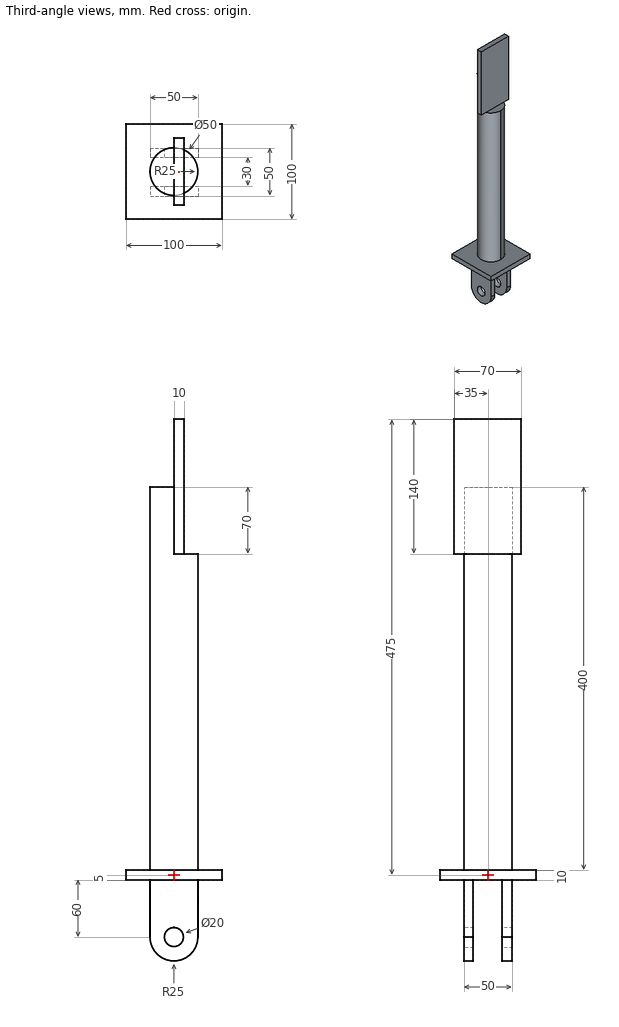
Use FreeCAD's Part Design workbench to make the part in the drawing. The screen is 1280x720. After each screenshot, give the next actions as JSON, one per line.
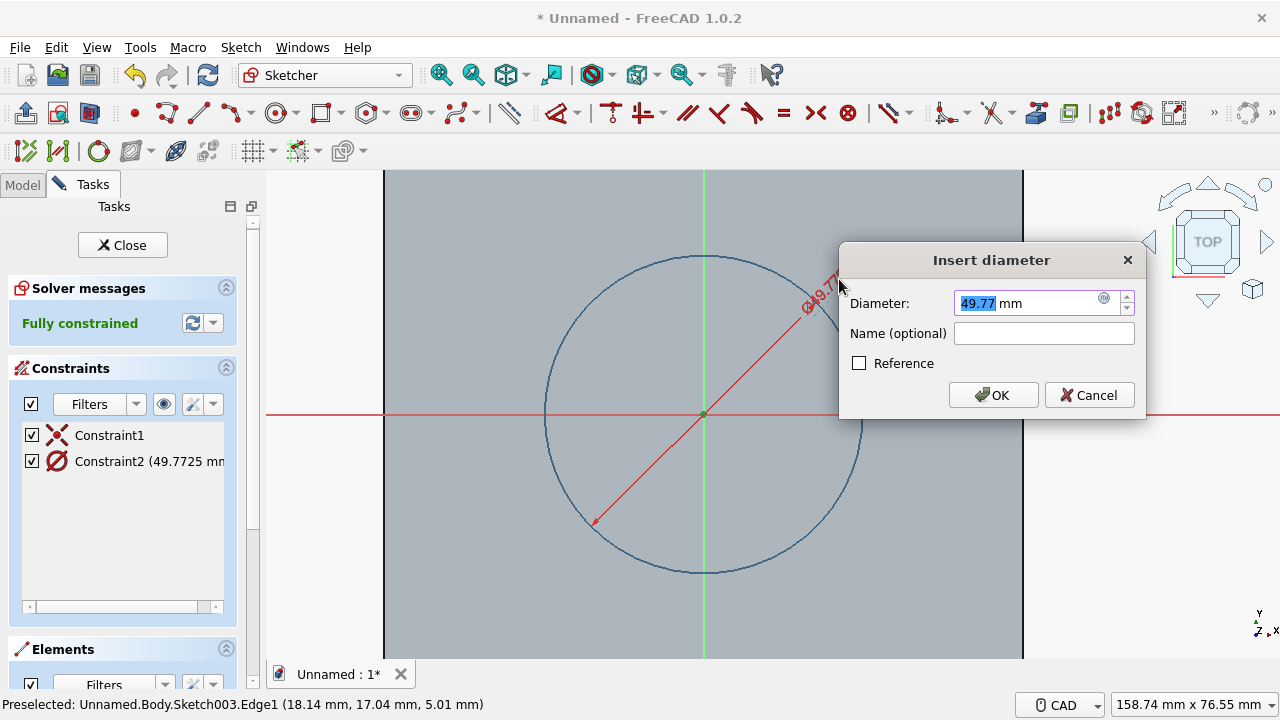
{"action": "type", "text": "50"}
{"action": "key", "text": "Return"}
{"action": "key", "text": "Escape"}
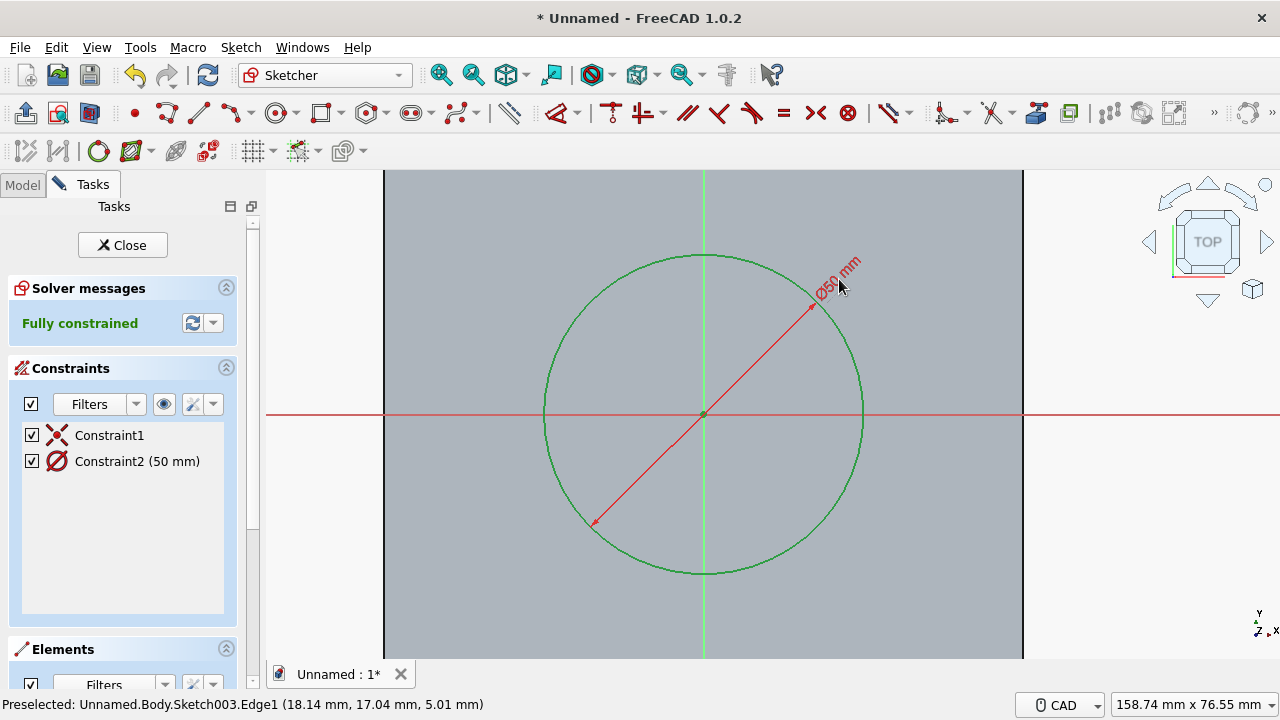
{"action": "left_click", "coordinate": [123, 245]}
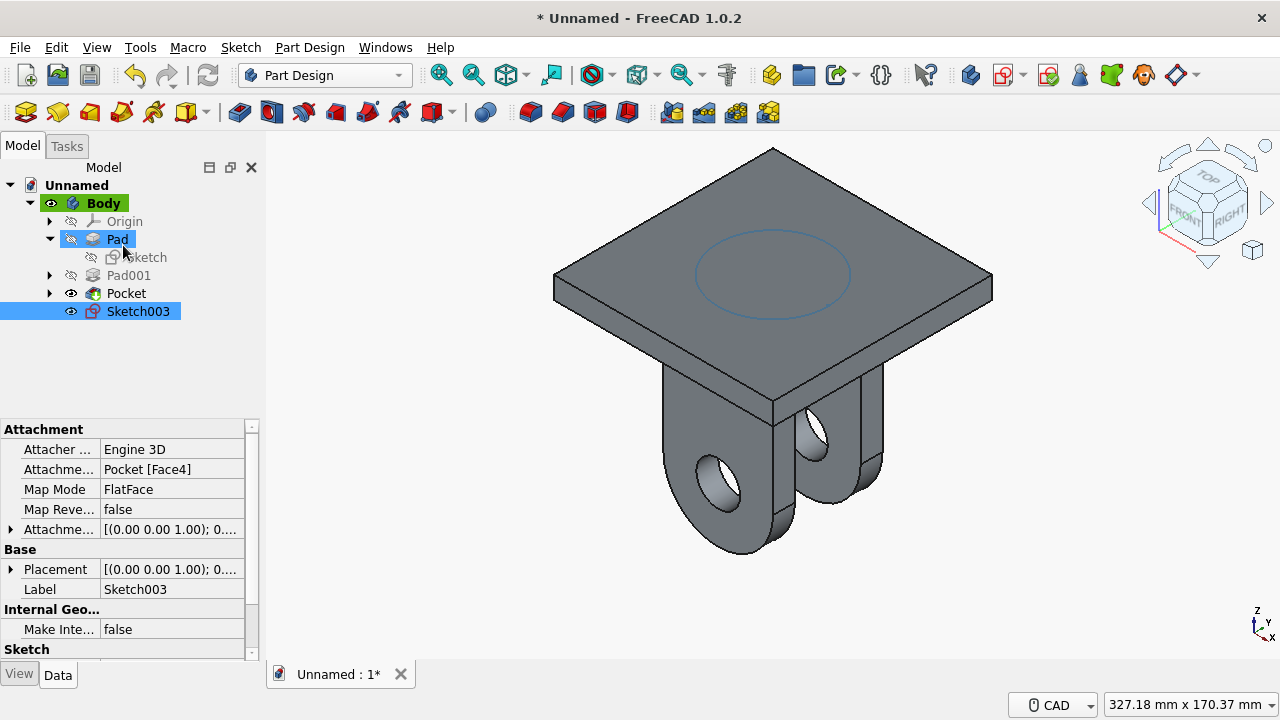
{"action": "left_click", "coordinate": [26, 112]}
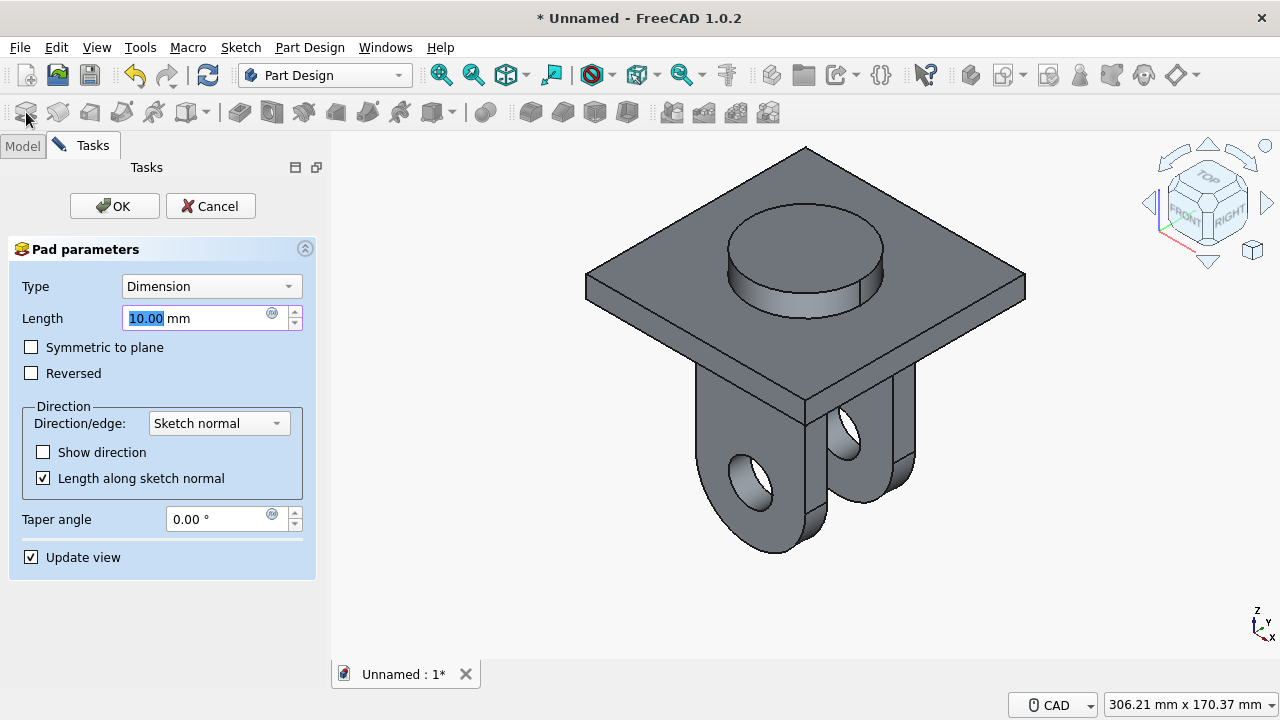
{"action": "type", "text": "400"}
{"action": "key", "text": "Tab"}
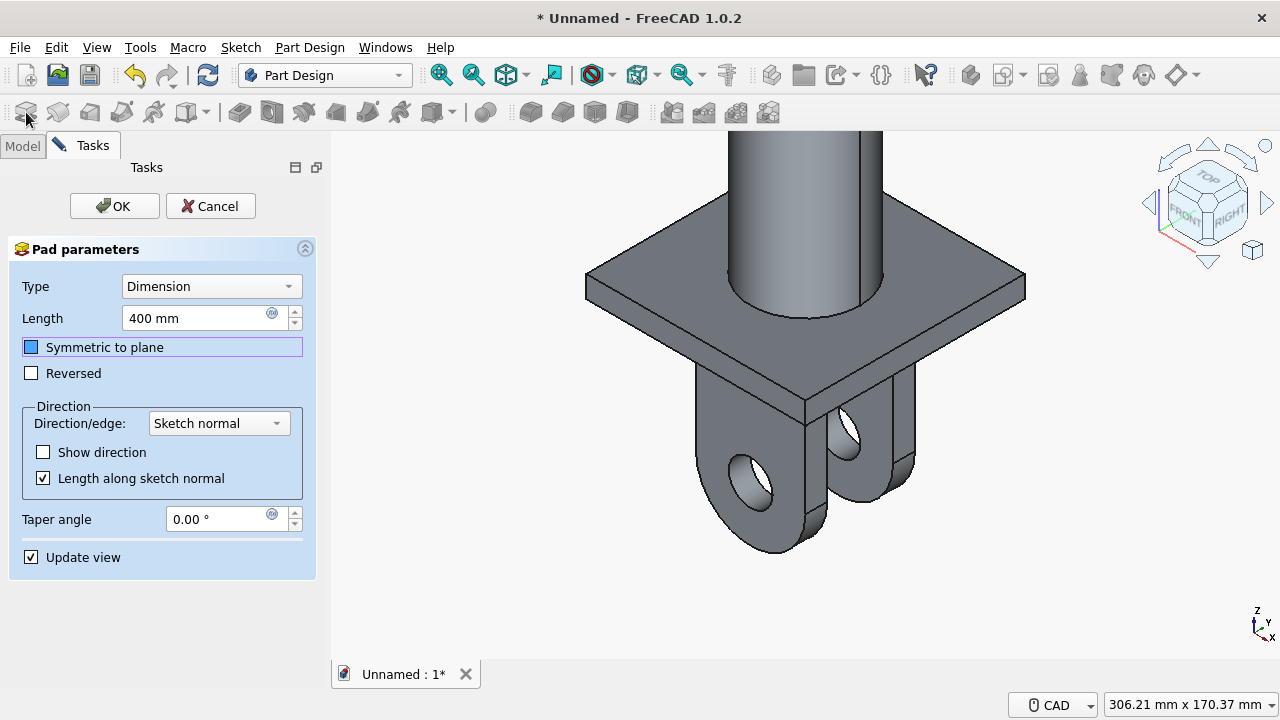
{"action": "left_click", "coordinate": [115, 206]}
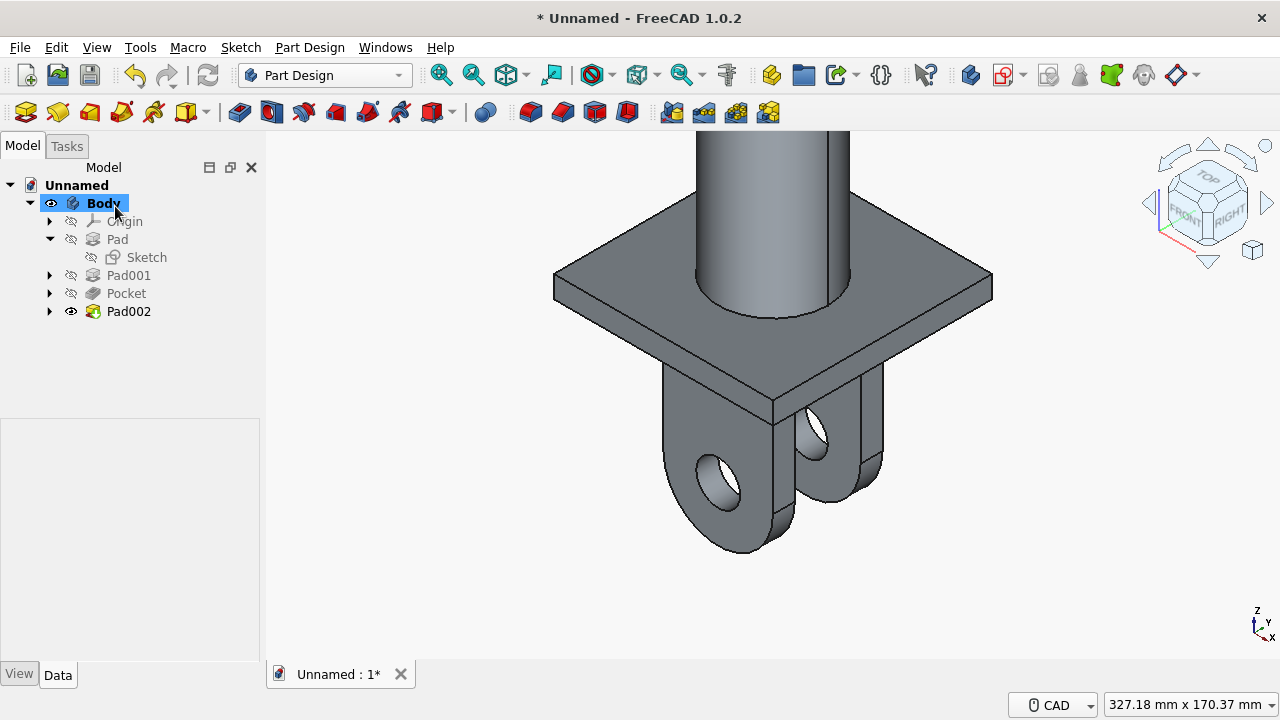
{"action": "key", "text": "v f"}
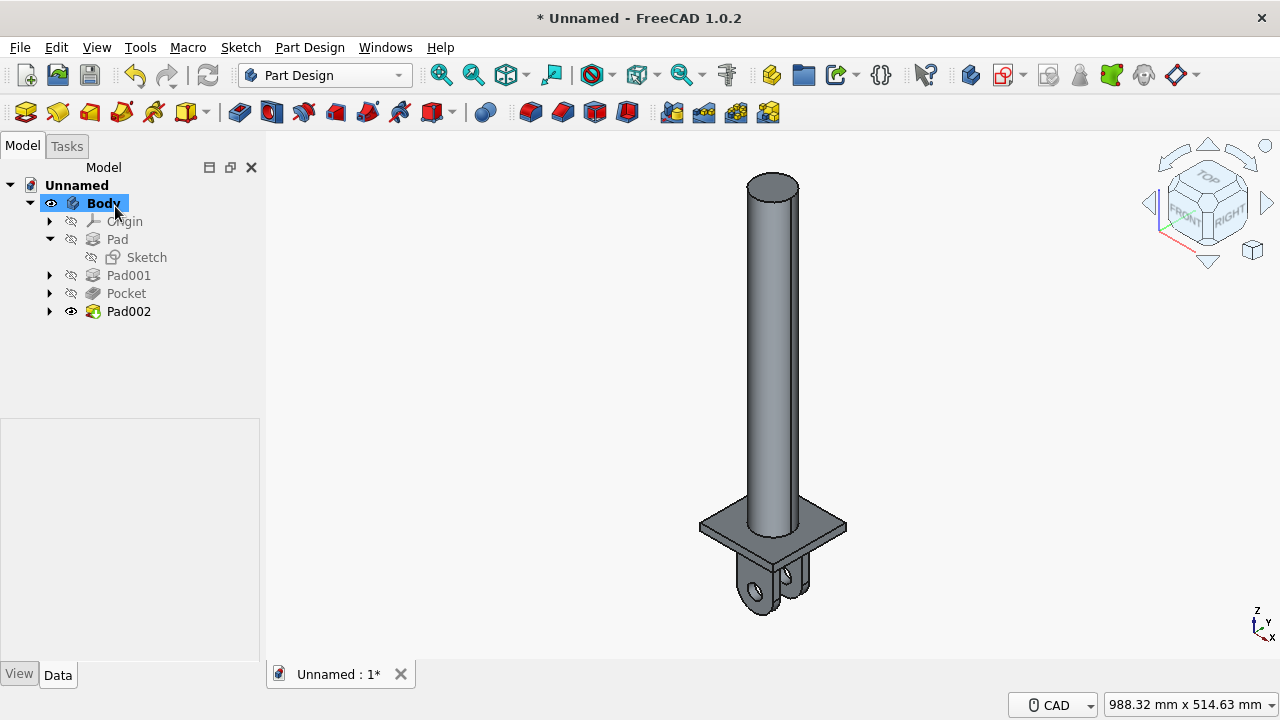
{"action": "left_click", "coordinate": [50, 221]}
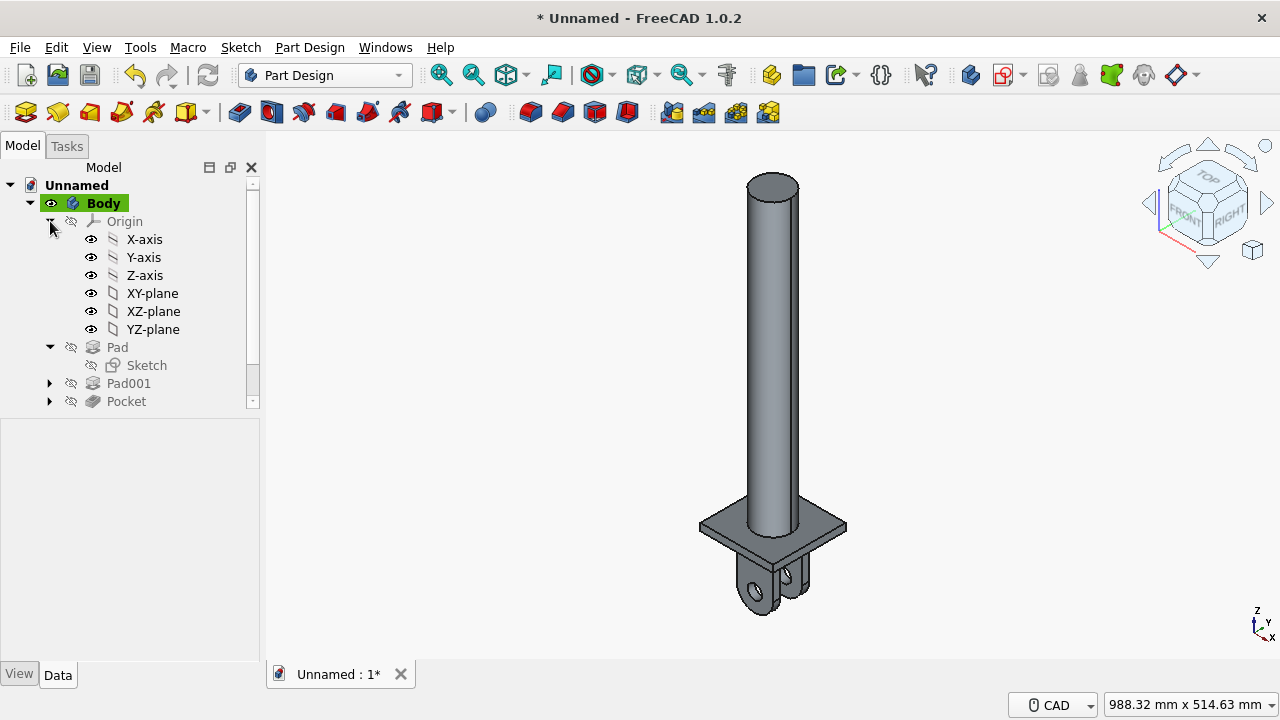
{"action": "left_click", "coordinate": [136, 293]}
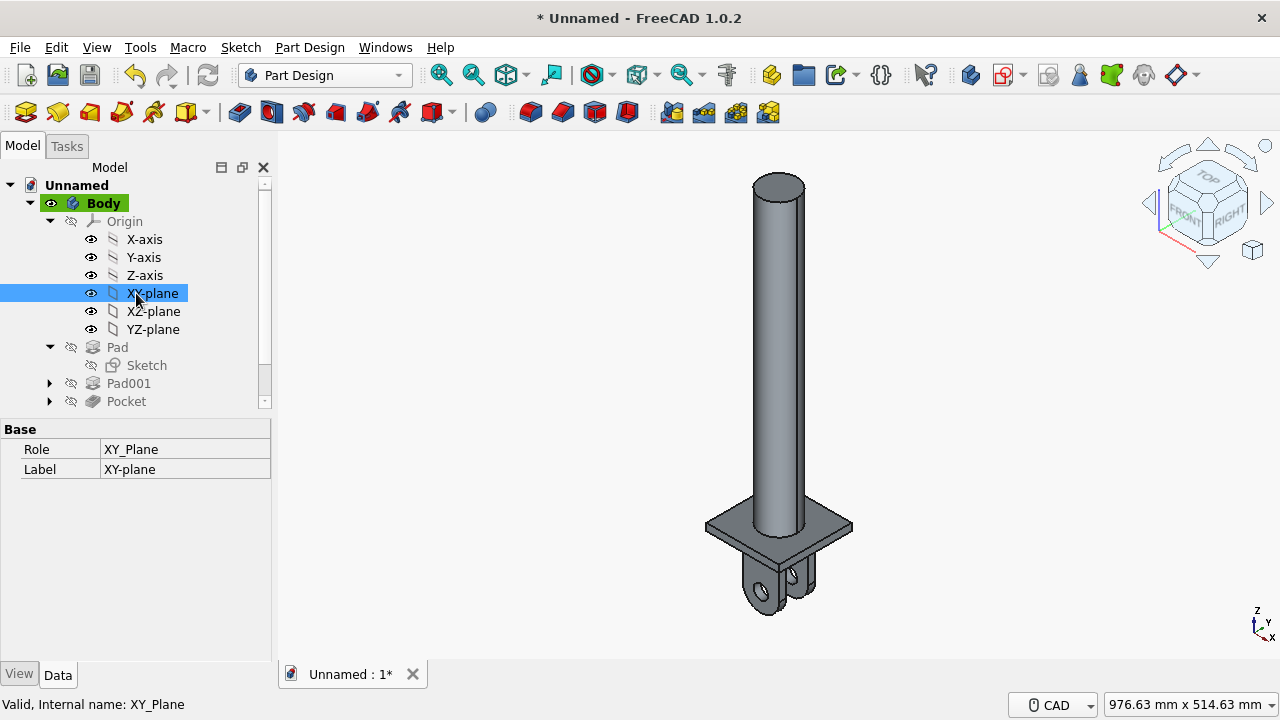
{"action": "left_click", "coordinate": [1176, 76]}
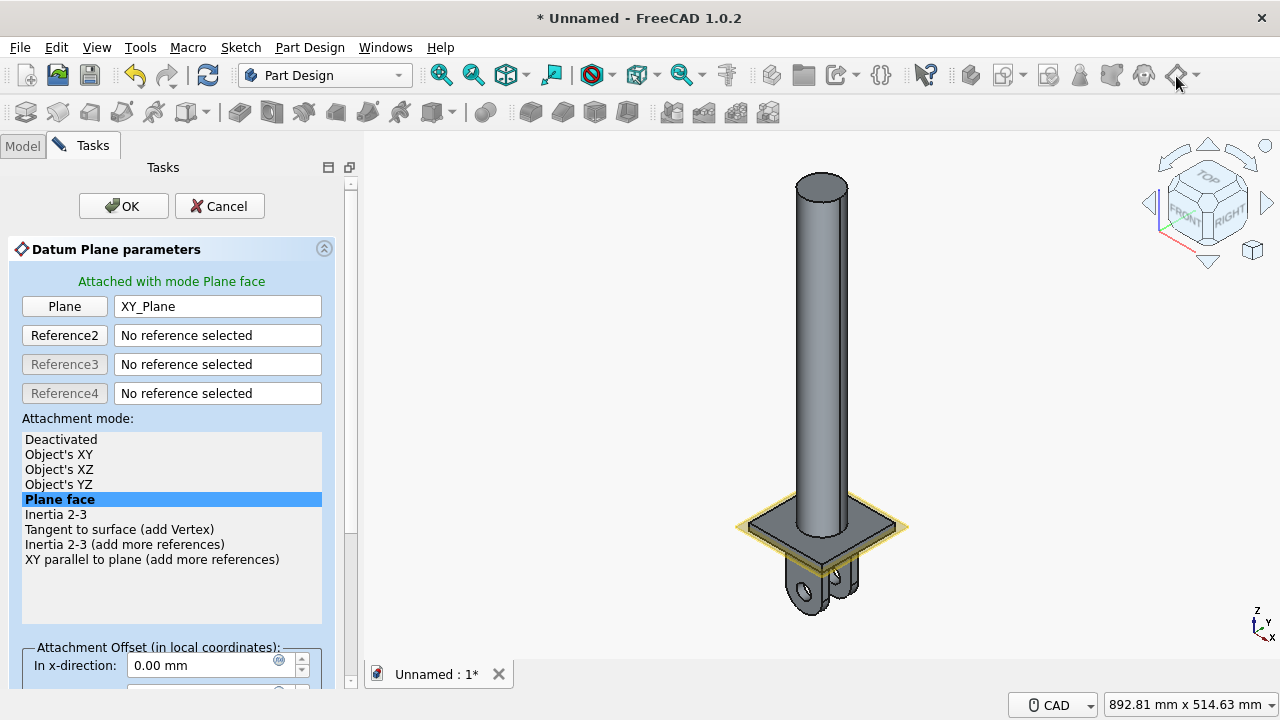
{"action": "scroll", "coordinate": [351, 432], "scroll_direction": "down", "scroll_amount": 2}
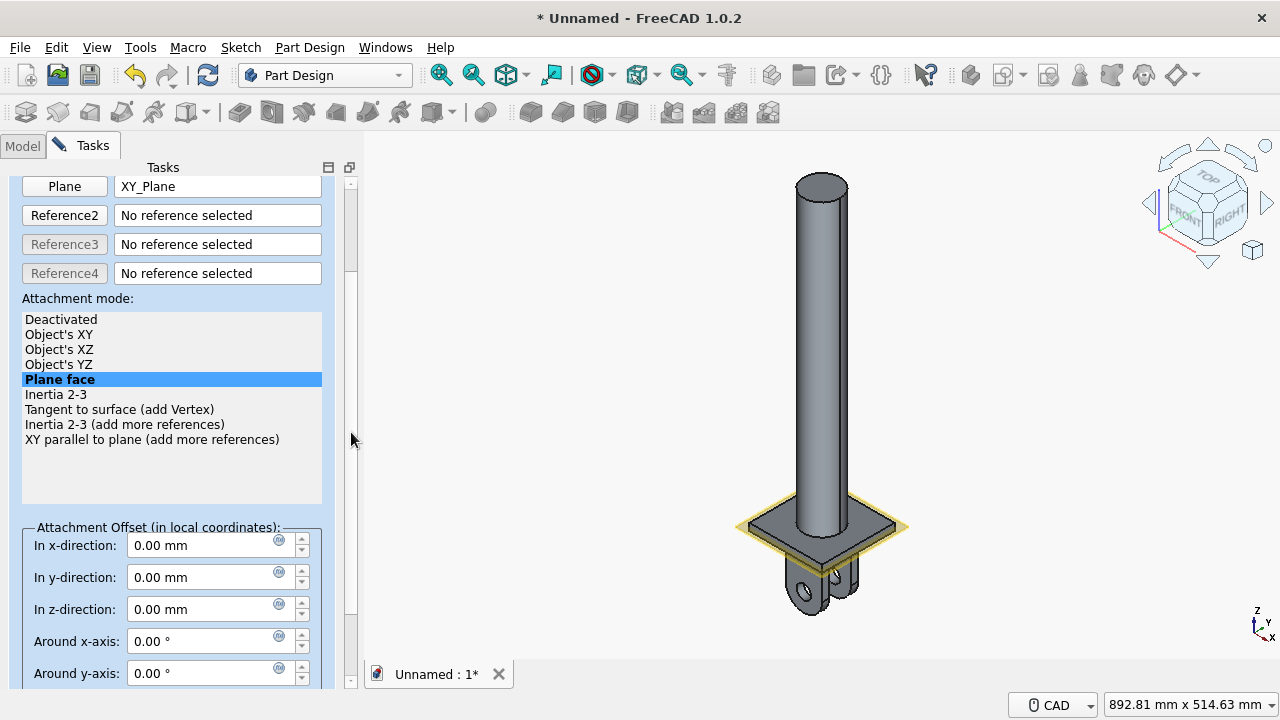
{"action": "triple_click", "coordinate": [210, 609]}